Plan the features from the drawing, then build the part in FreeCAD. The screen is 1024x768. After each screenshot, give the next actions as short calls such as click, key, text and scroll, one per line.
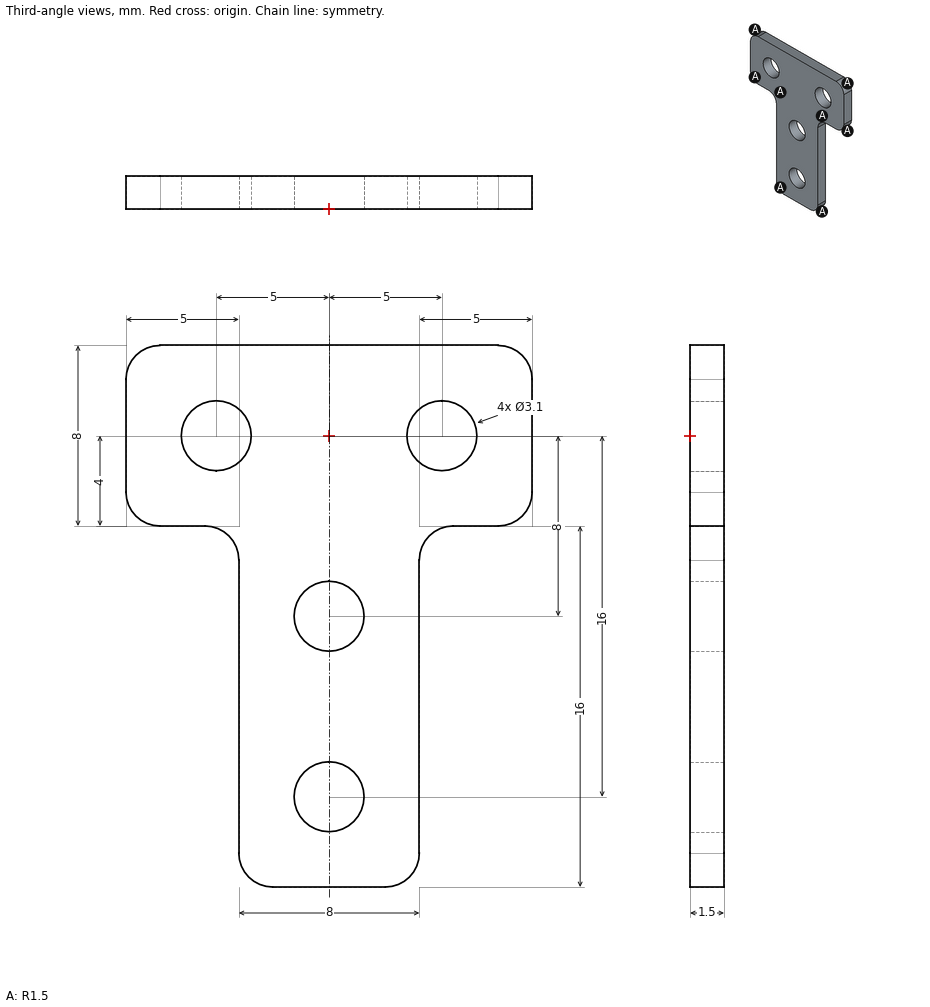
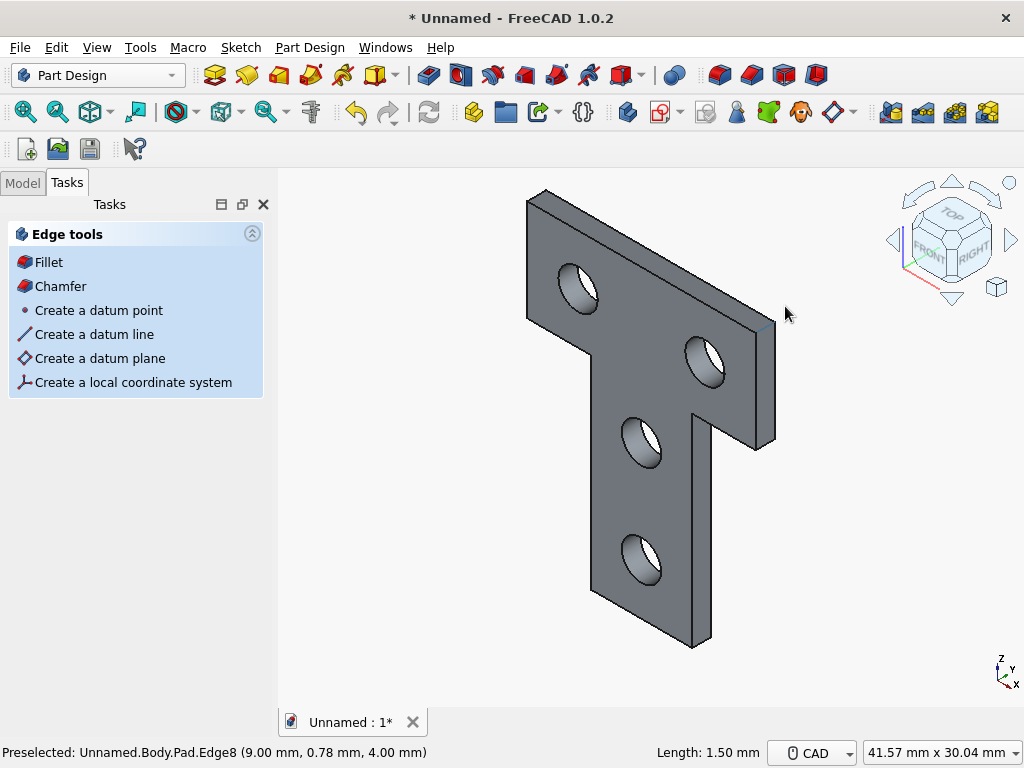
key(2)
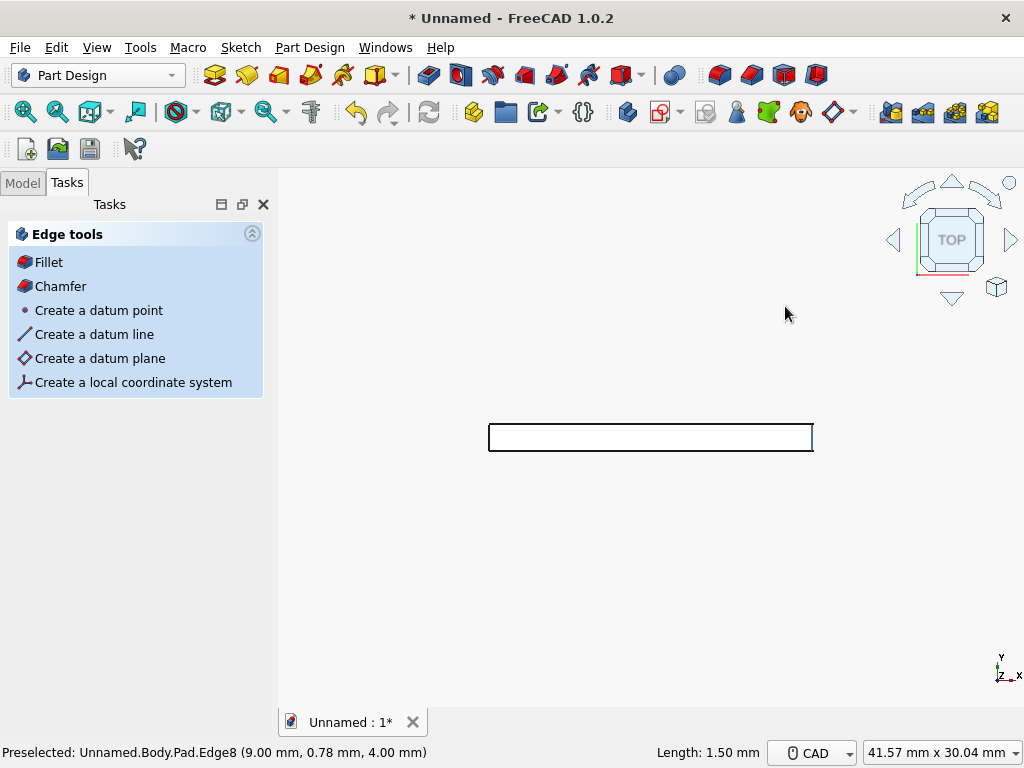
click(26, 112)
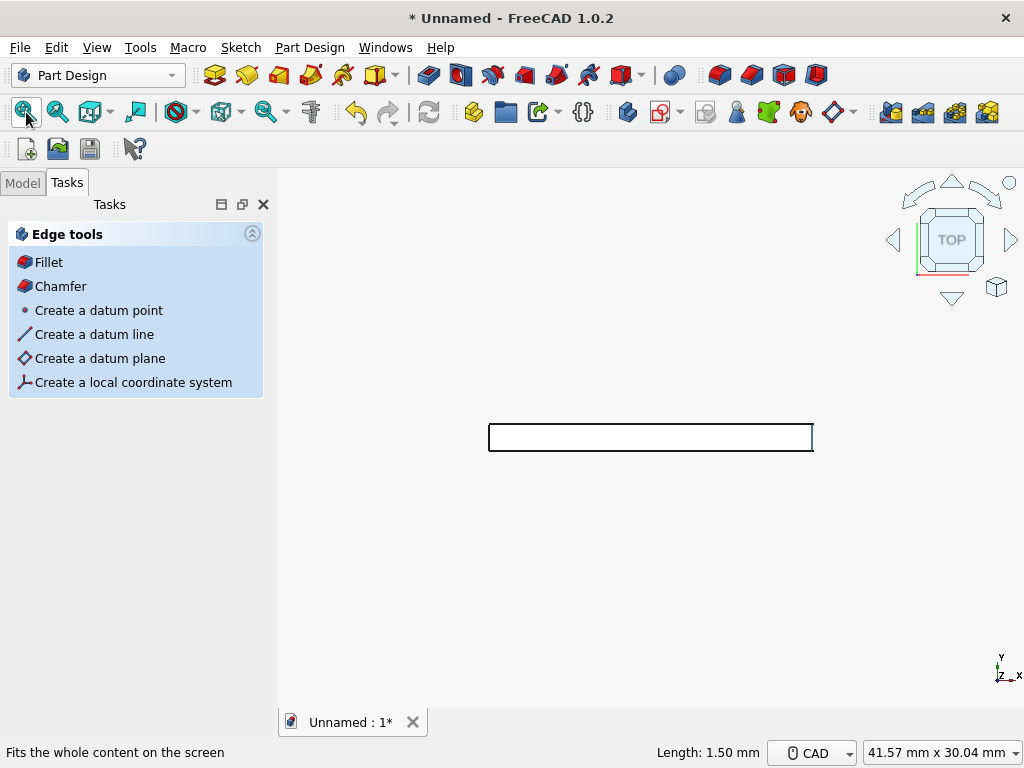
click(490, 437, ctrl)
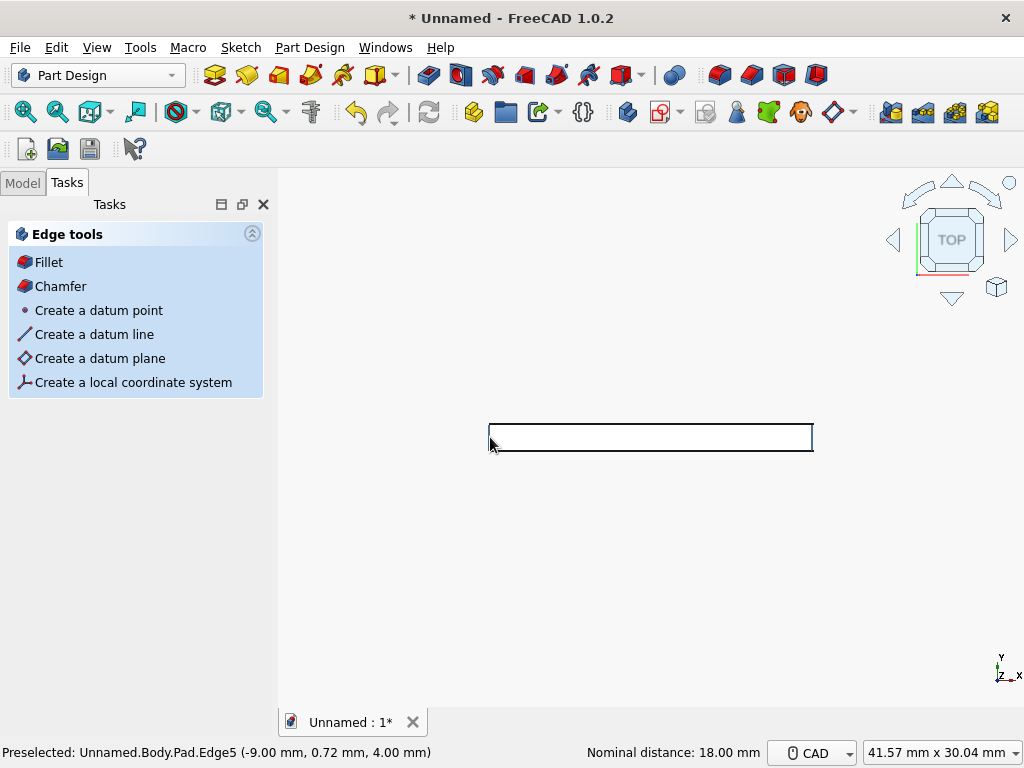
key(1)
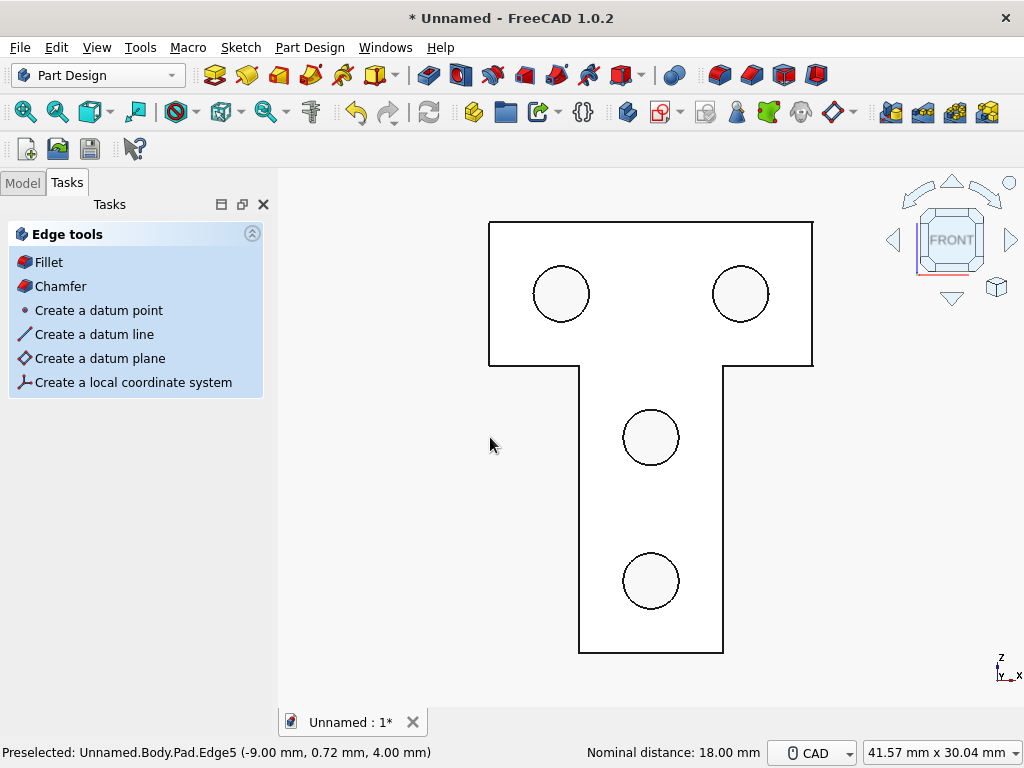
key(3)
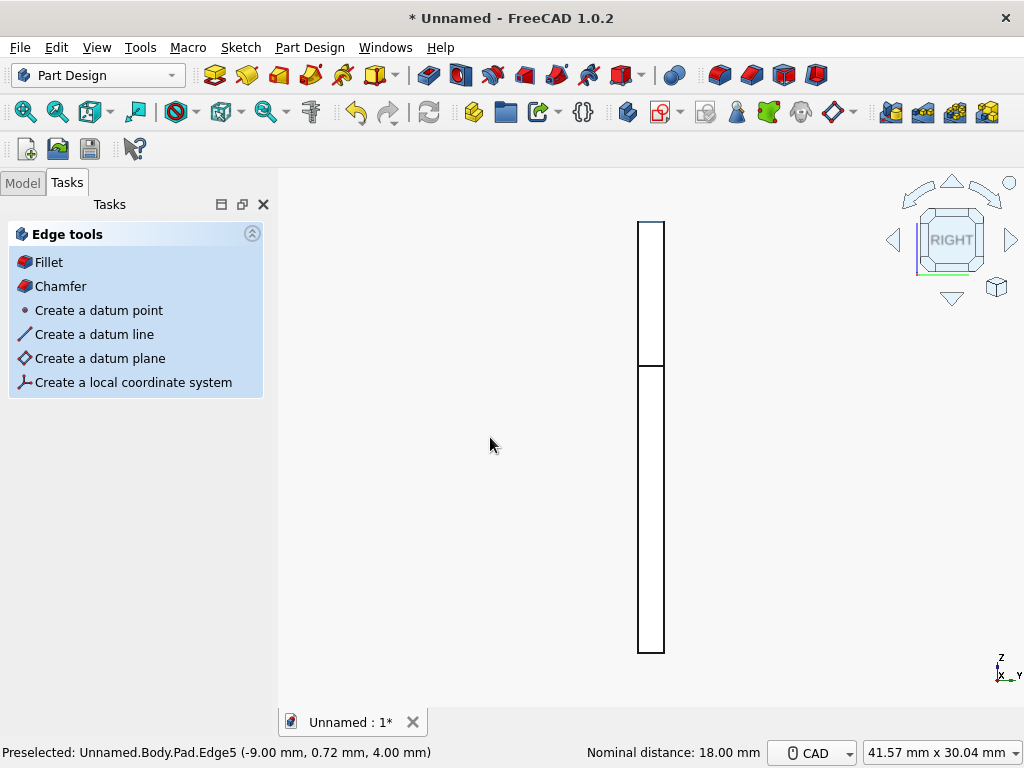
click(651, 365, ctrl)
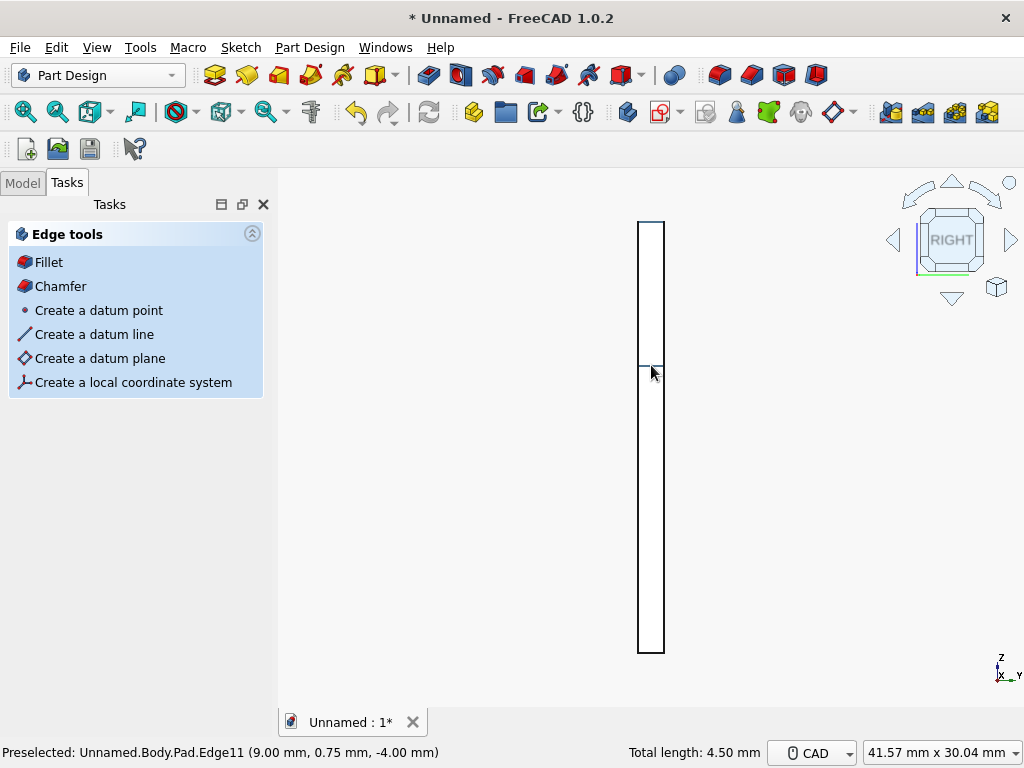
click(651, 652, ctrl)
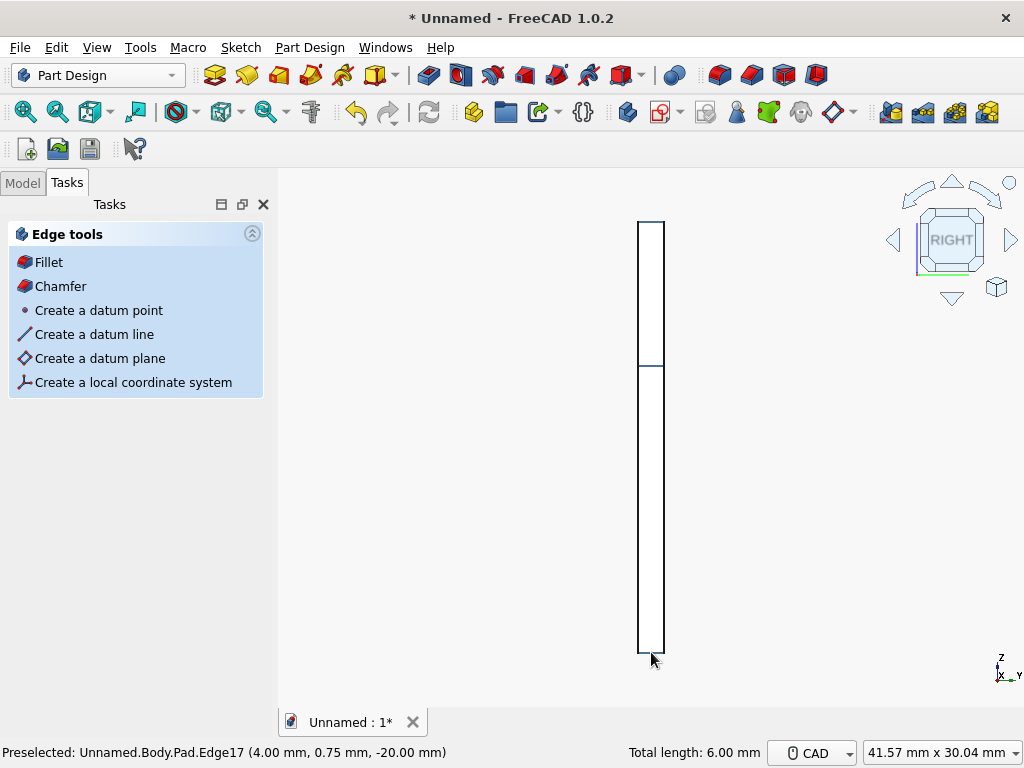
key(5)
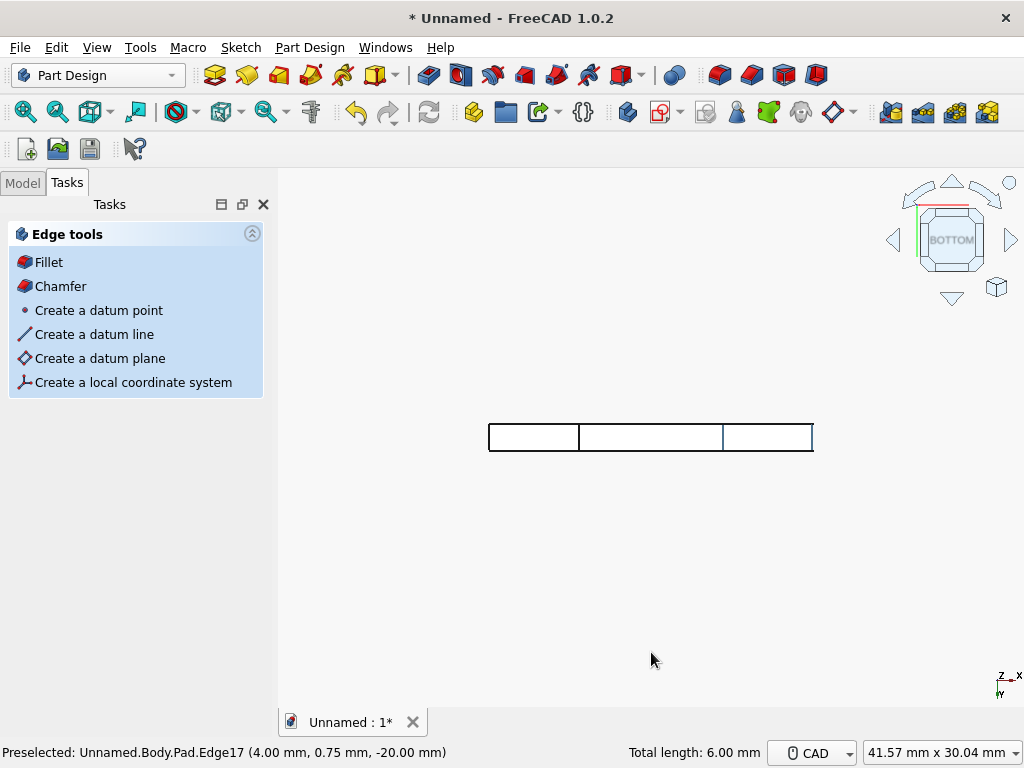
click(26, 112)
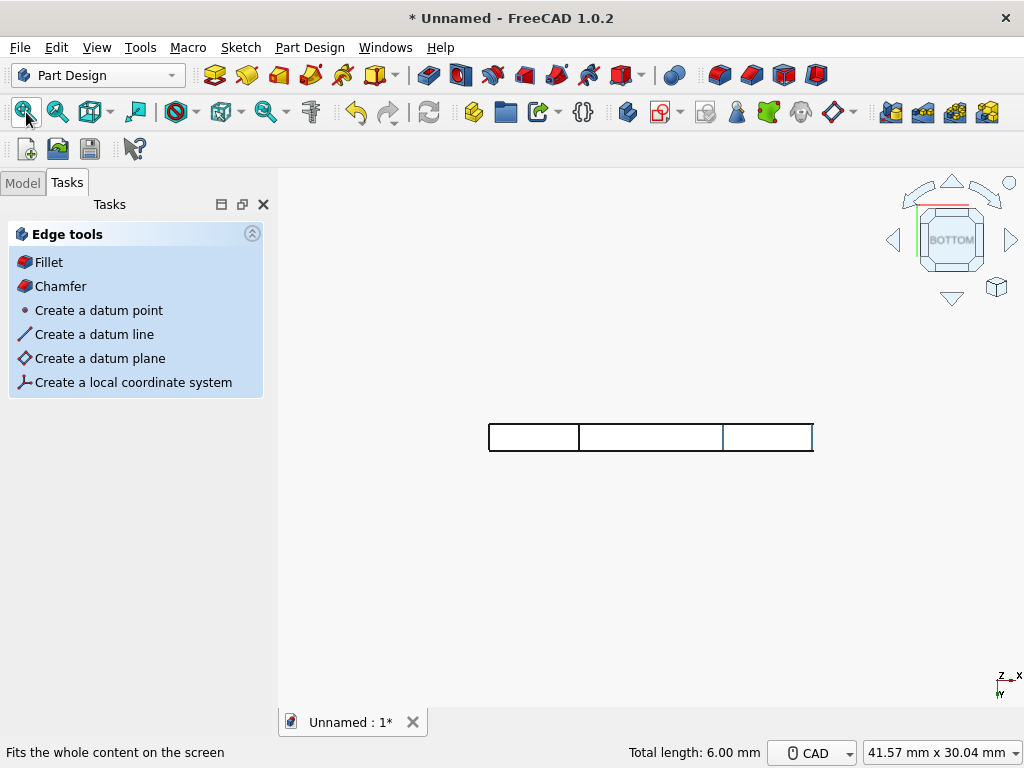
click(490, 436, ctrl)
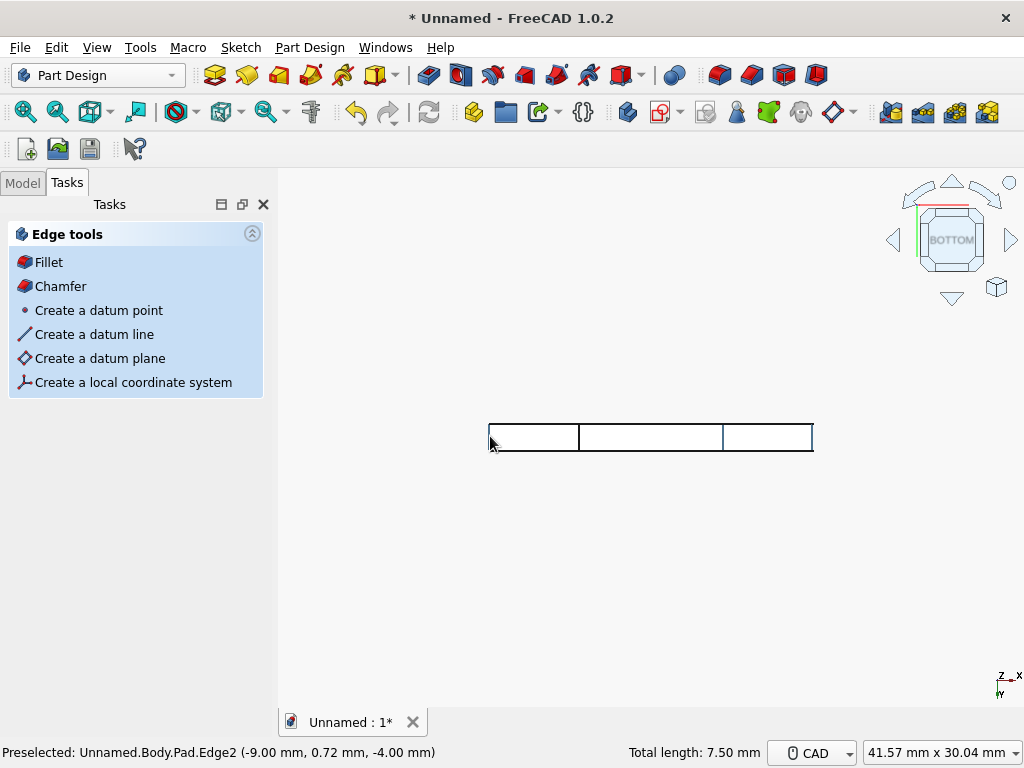
click(579, 436, ctrl)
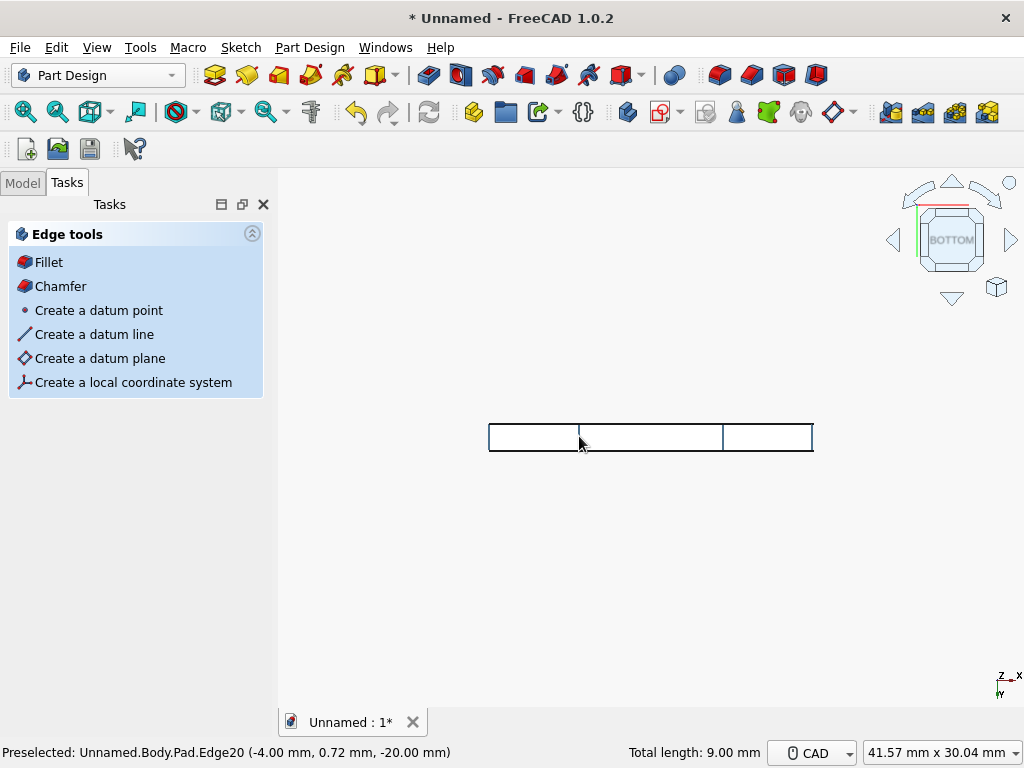
key(4)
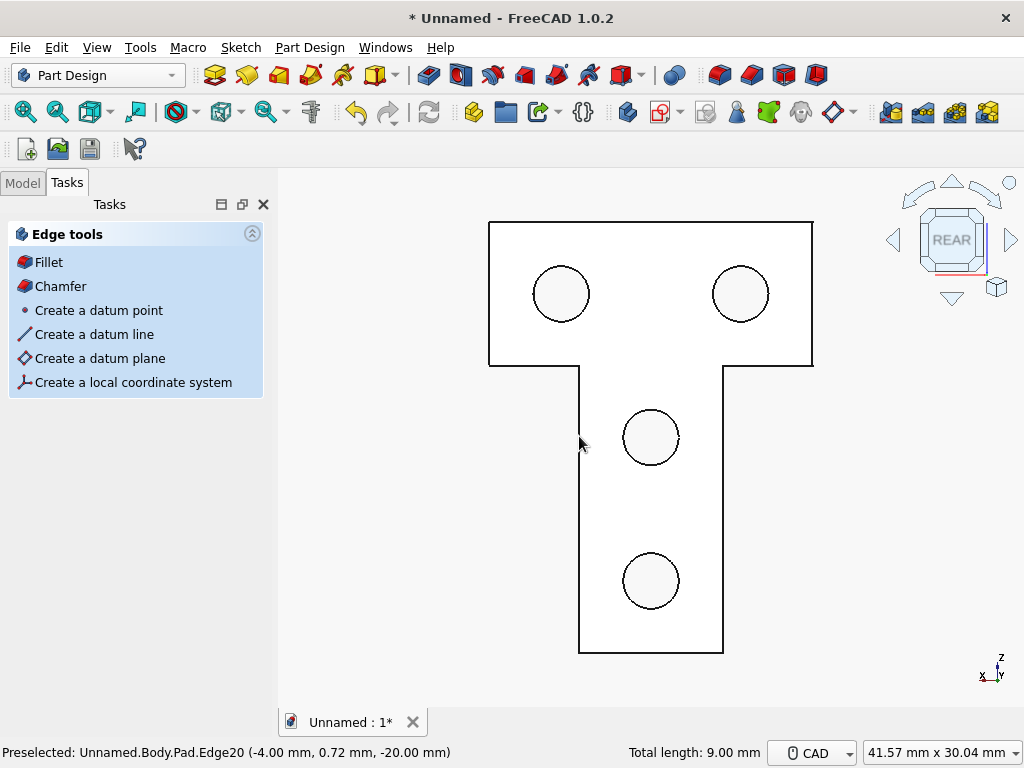
key(6)